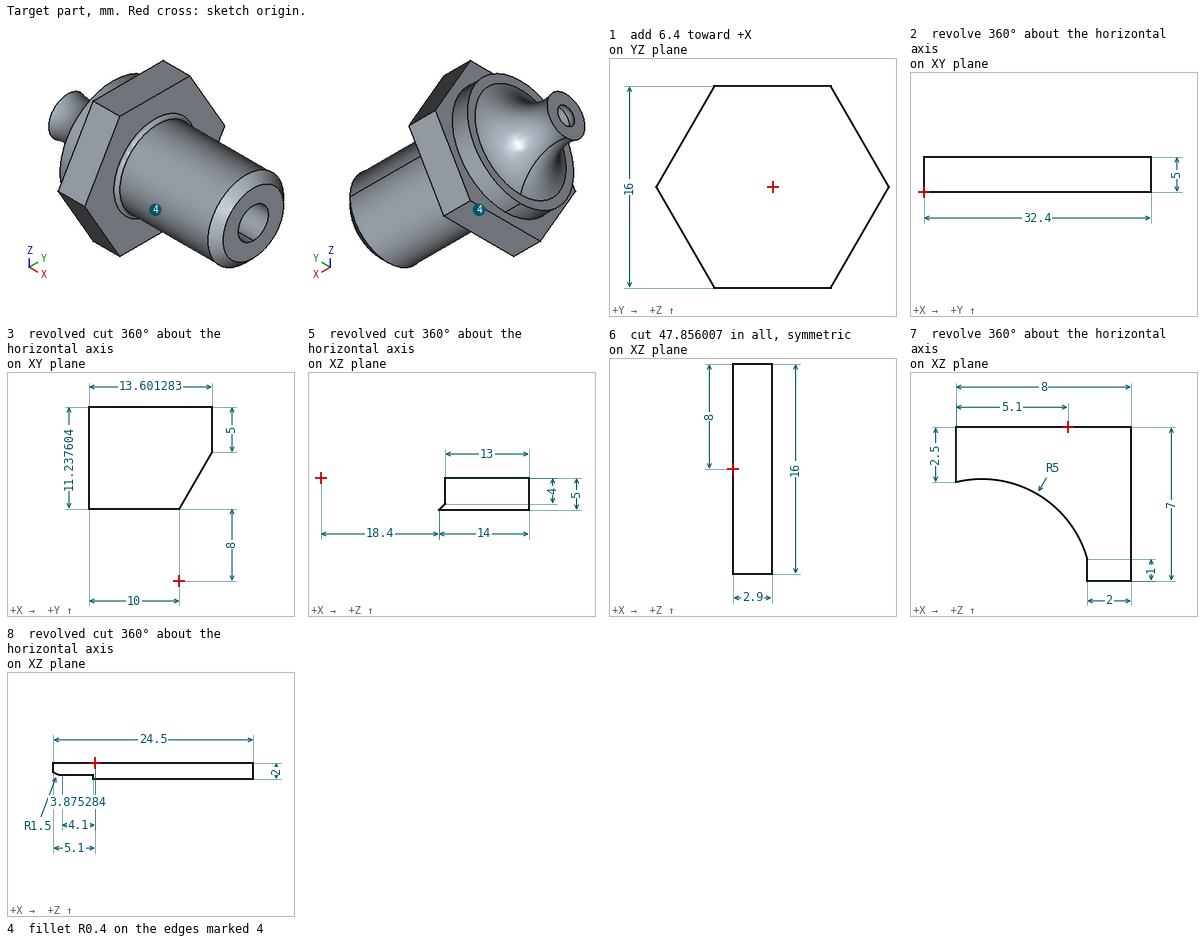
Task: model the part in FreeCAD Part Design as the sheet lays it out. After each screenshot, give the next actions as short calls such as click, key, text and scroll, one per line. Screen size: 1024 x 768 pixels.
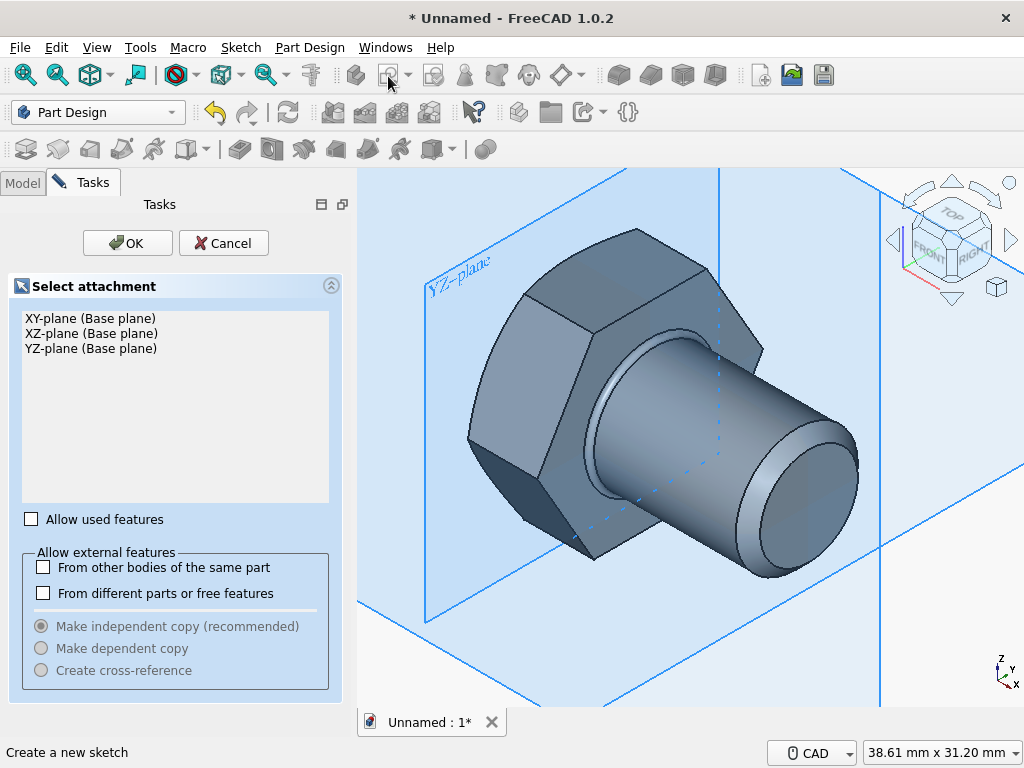
click(82, 334)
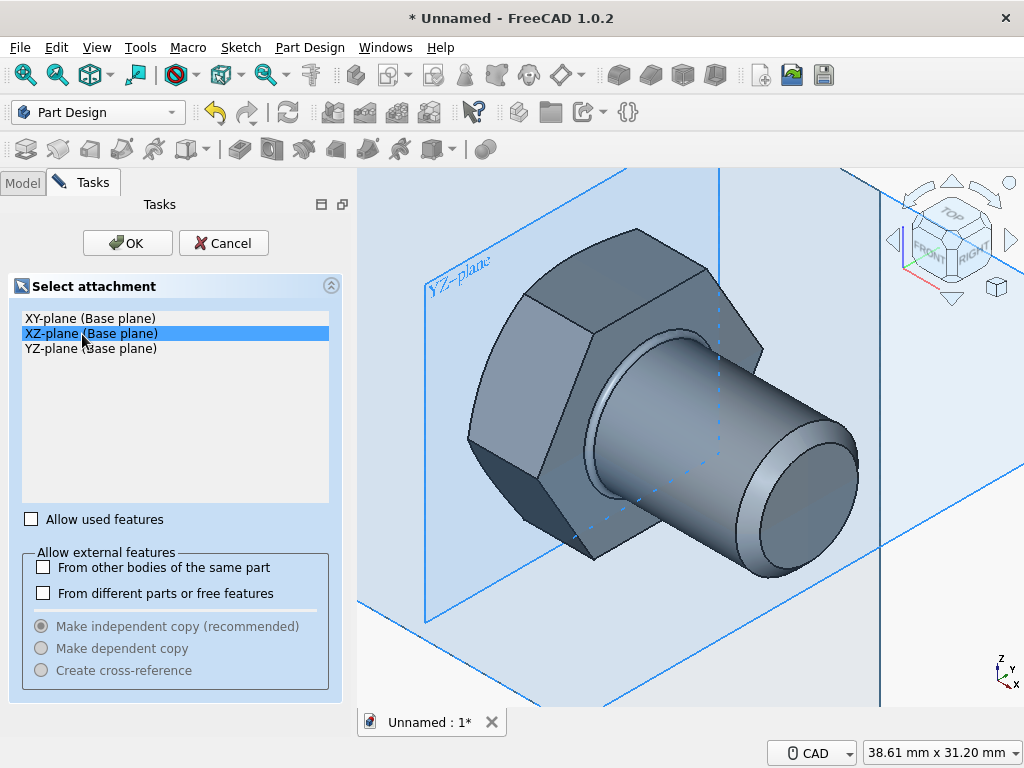
click(128, 243)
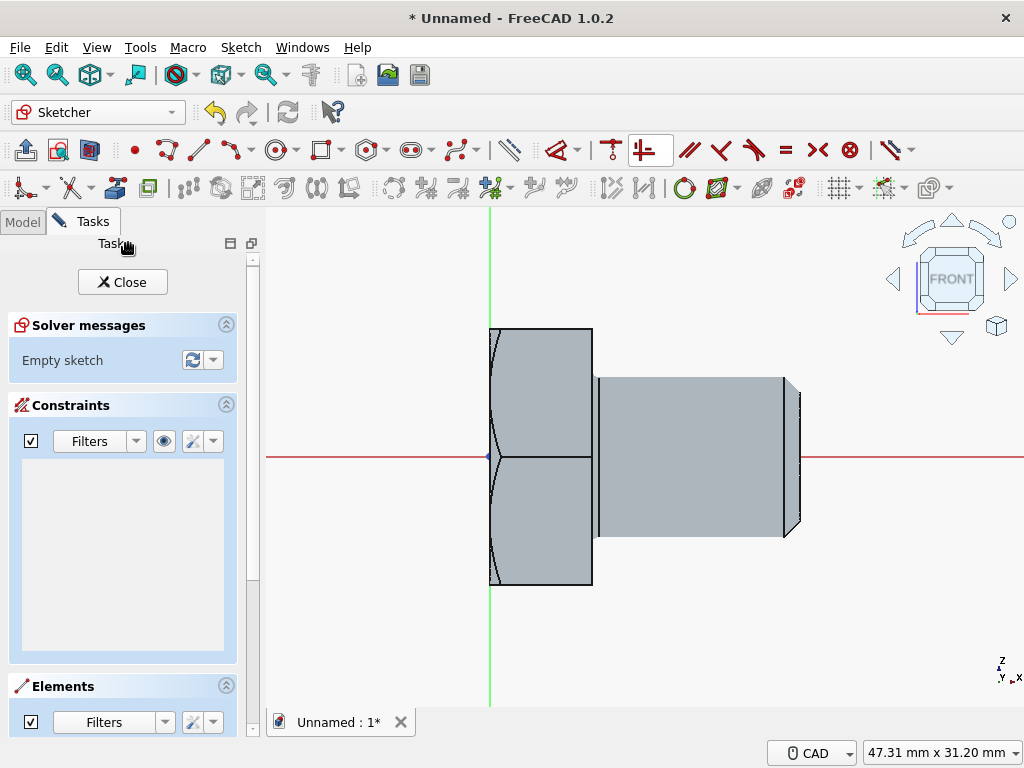
click(90, 150)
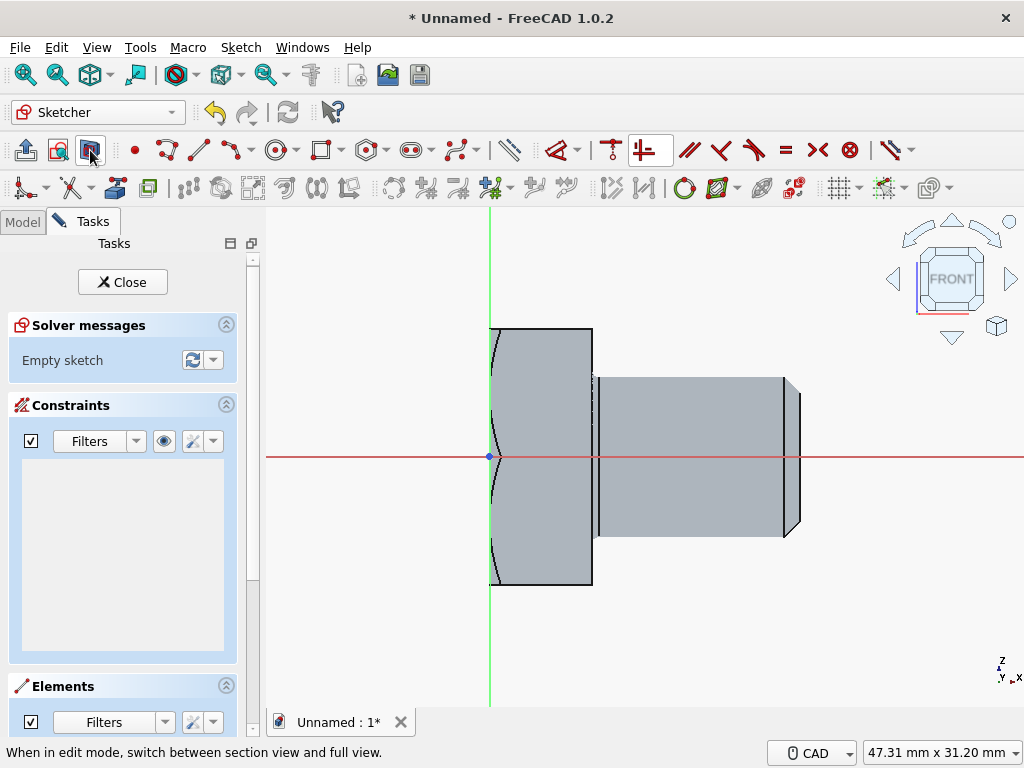
click(322, 150)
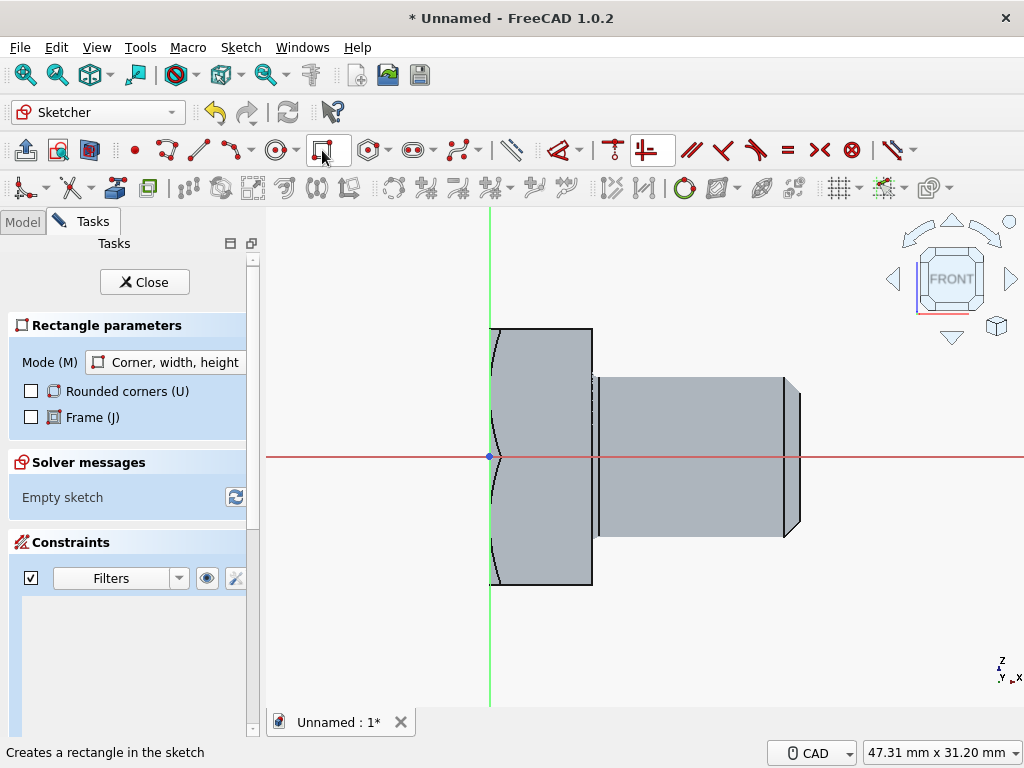
click(490, 329)
move(536, 585)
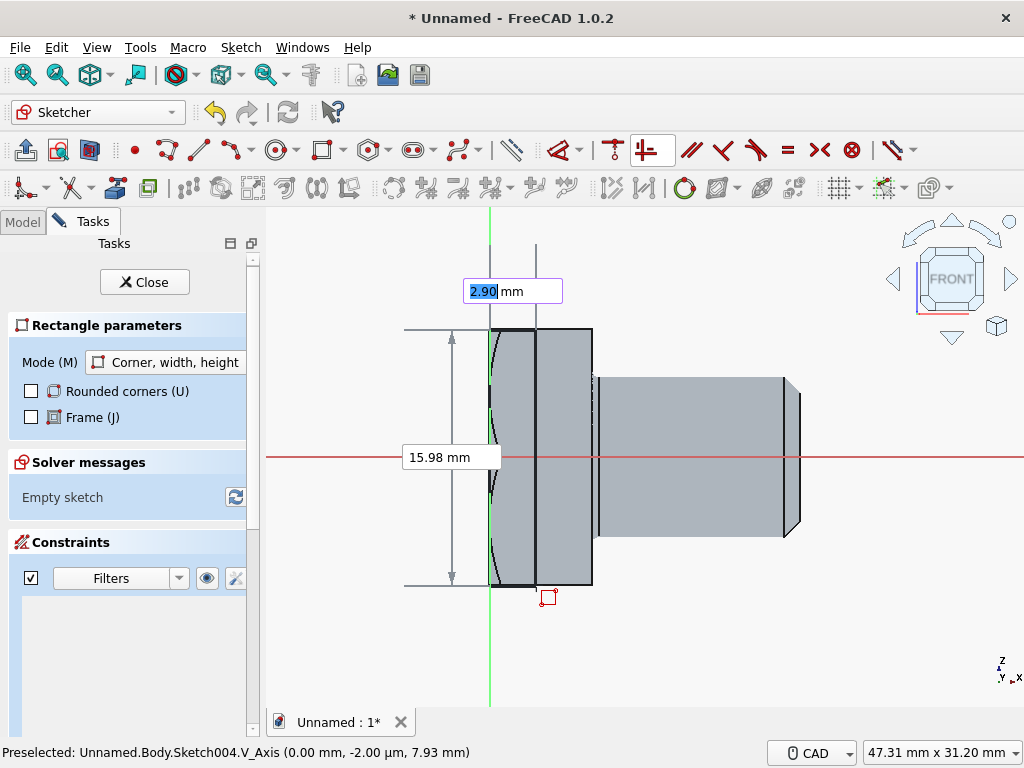
text(2.9)
key(Tab)
text(16)
key(Return)
key(Escape)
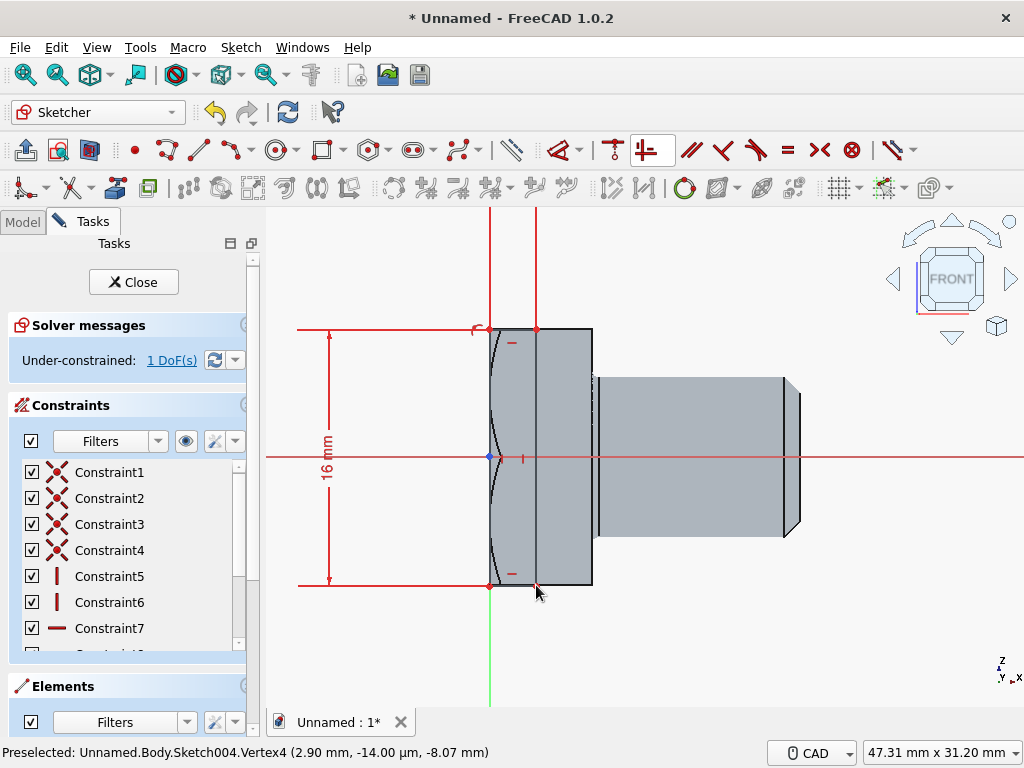
click(558, 150)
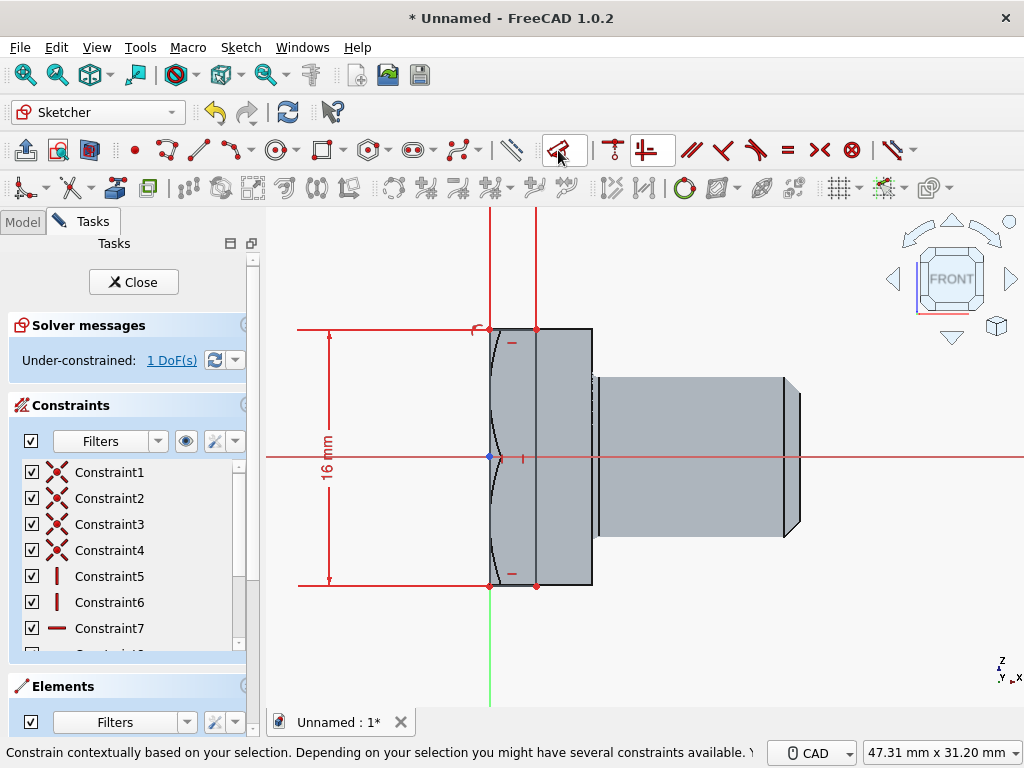
click(490, 330)
click(456, 394)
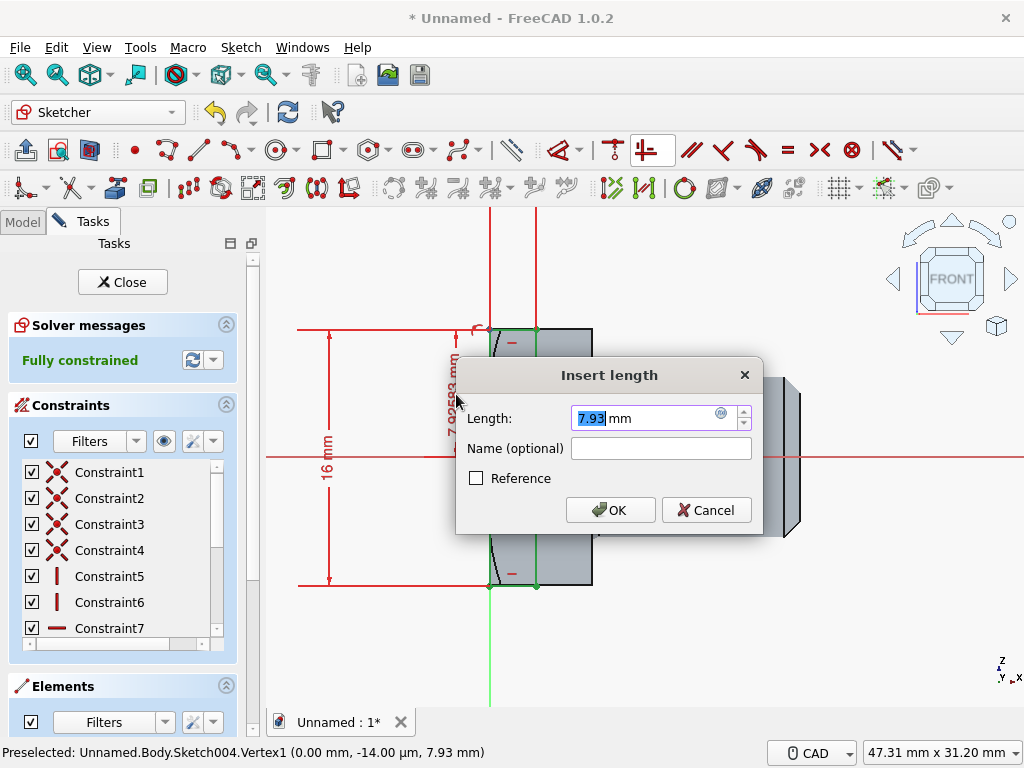
text(8)
key(Return)
key(Escape)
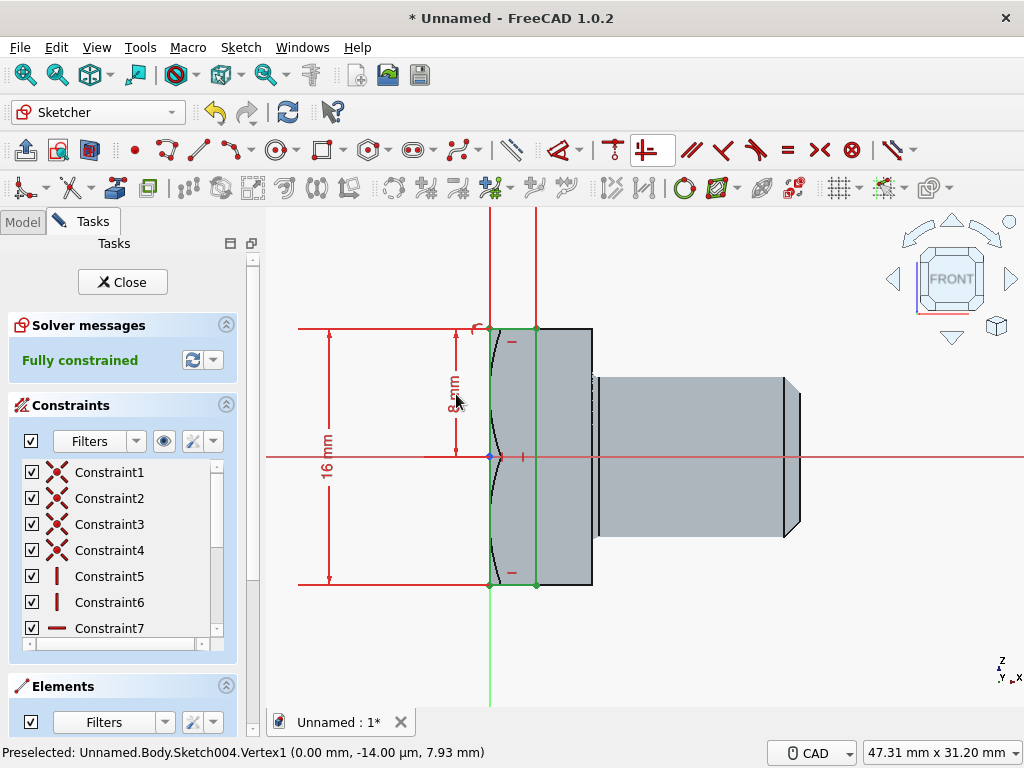
click(123, 282)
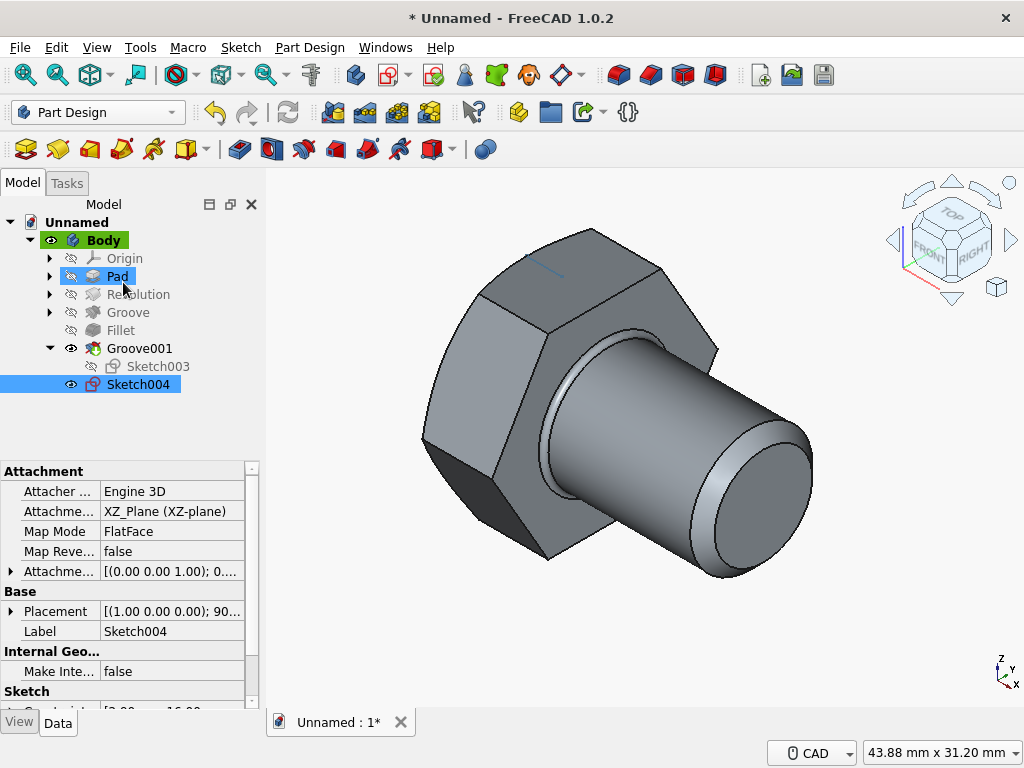
click(240, 150)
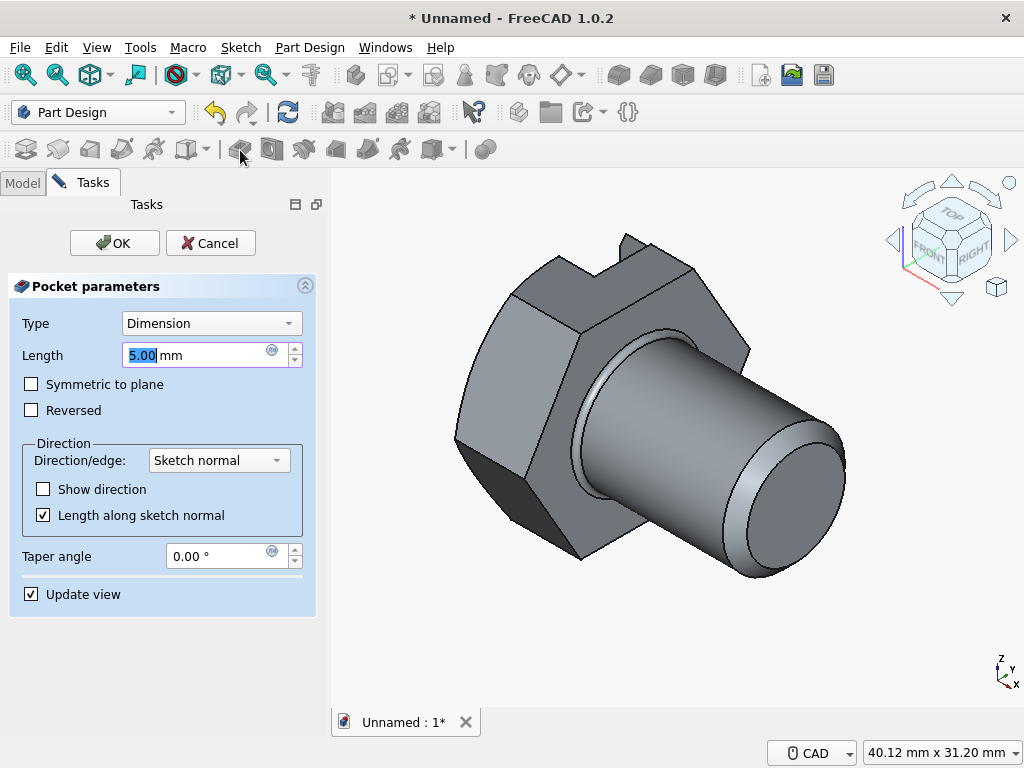
text(47.856007)
key(Tab)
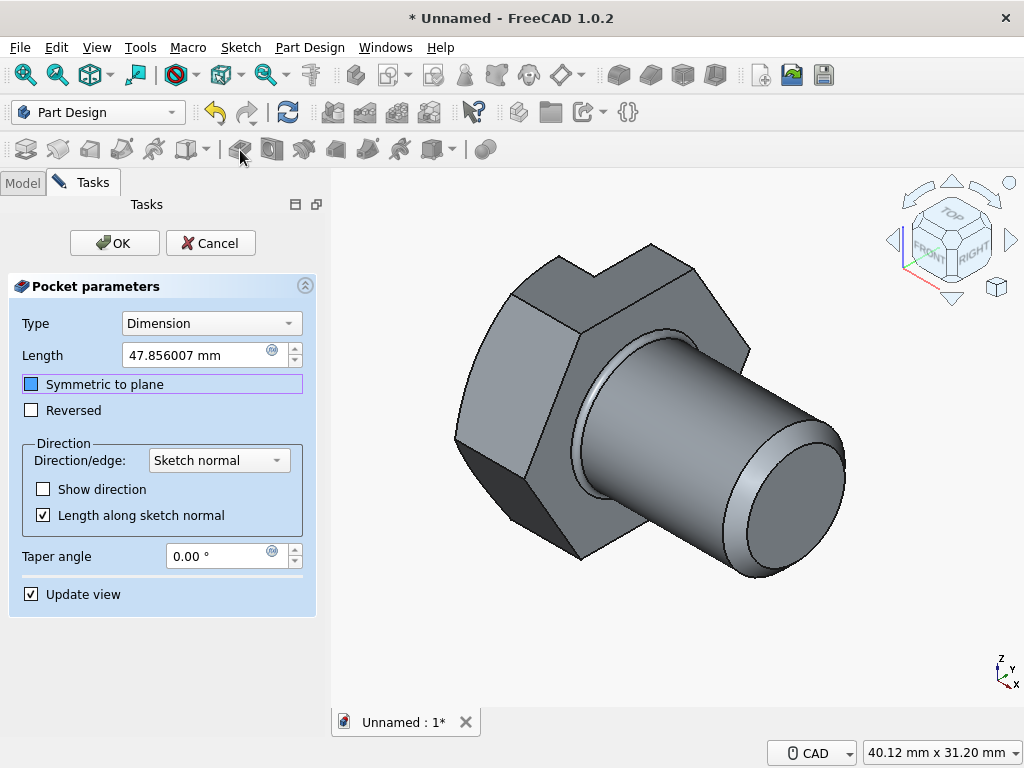
click(30, 384)